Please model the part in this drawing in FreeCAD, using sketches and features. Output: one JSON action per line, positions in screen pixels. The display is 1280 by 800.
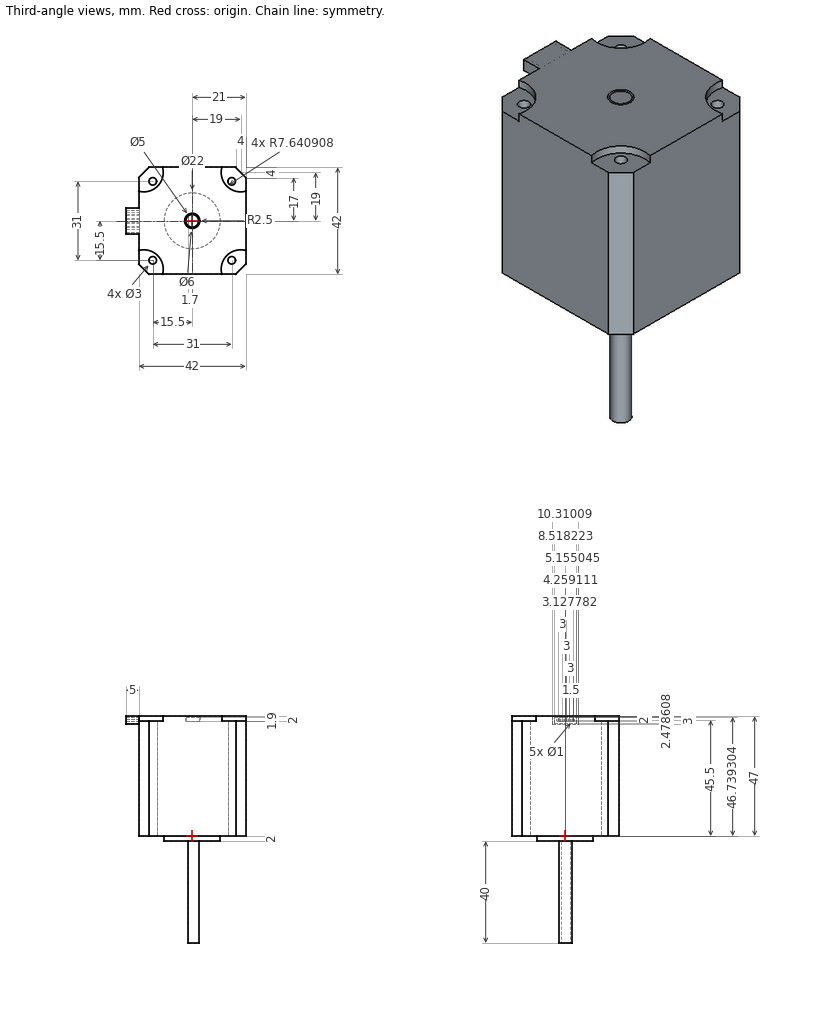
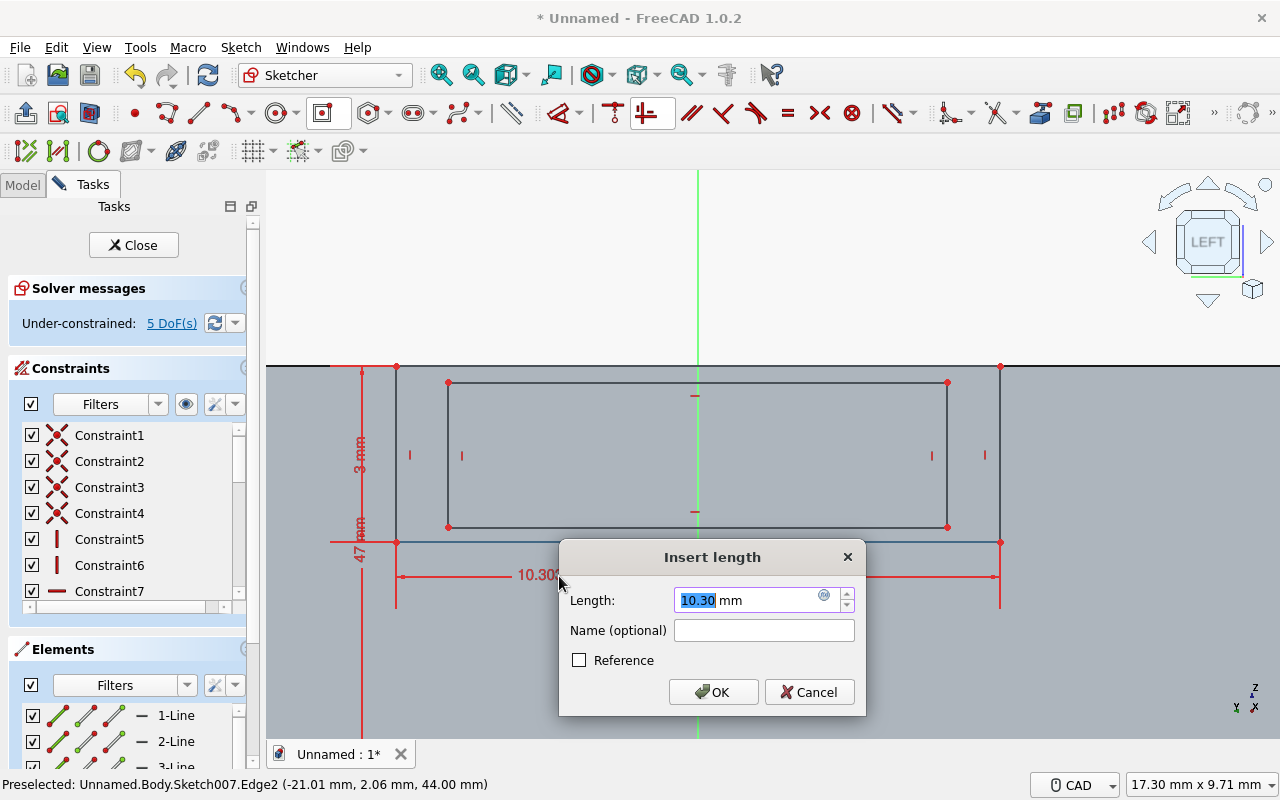
{"action": "type", "text": "10.31009"}
{"action": "key", "text": "Return"}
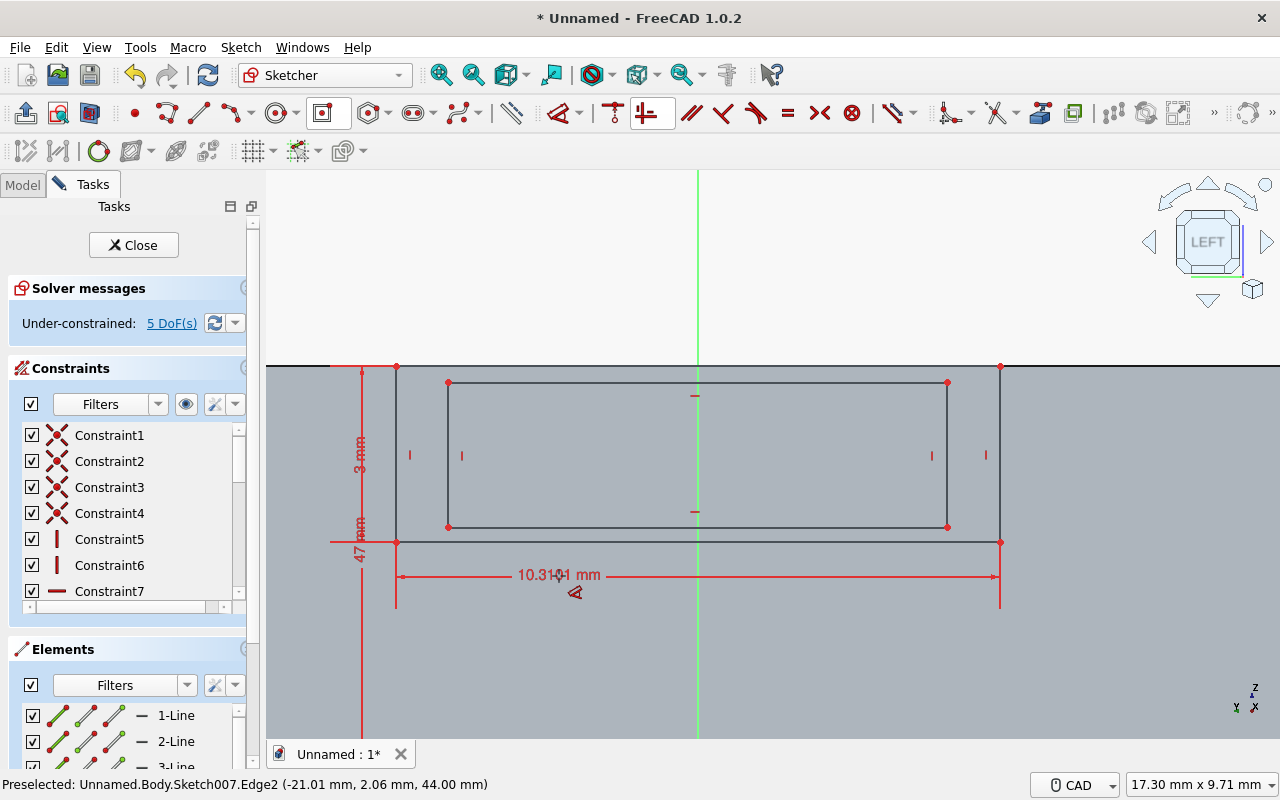
{"action": "left_click", "coordinate": [448, 427]}
{"action": "left_click", "coordinate": [414, 422]}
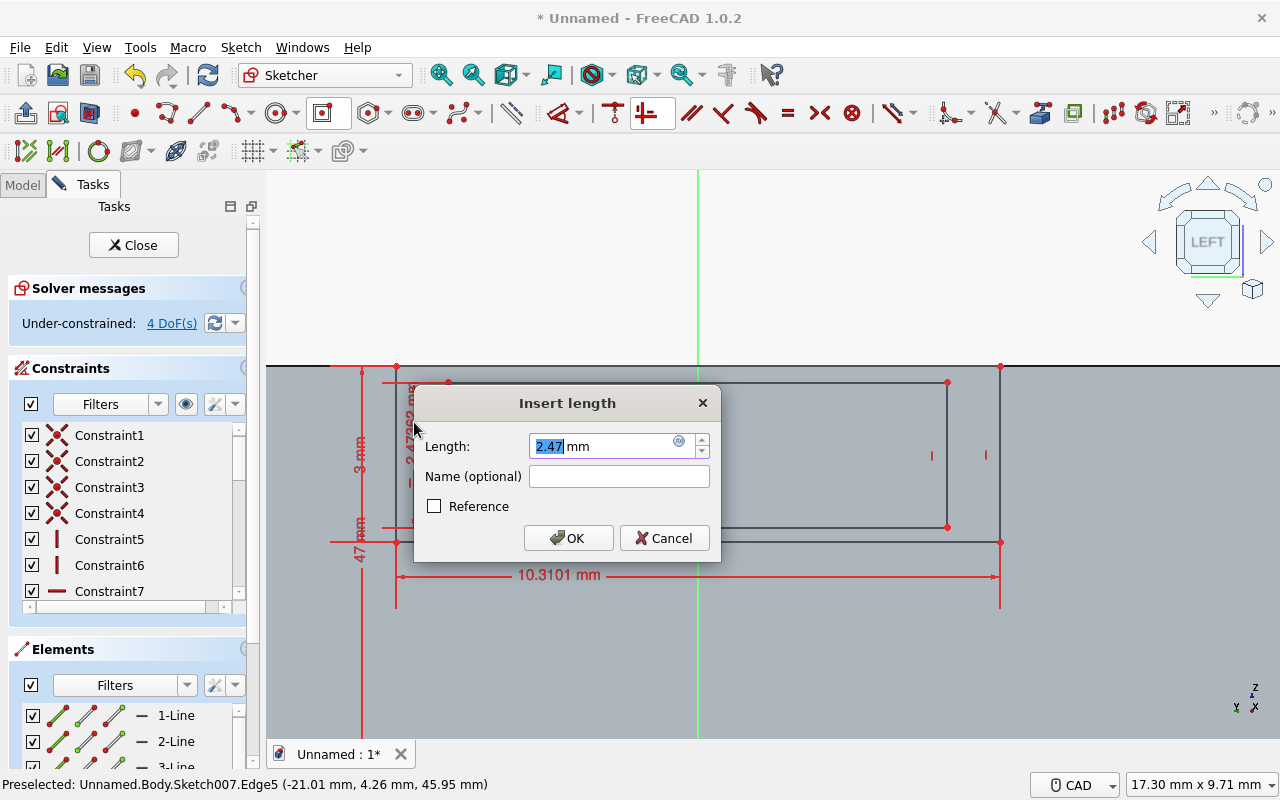
{"action": "type", "text": "2.478608"}
{"action": "key", "text": "Return"}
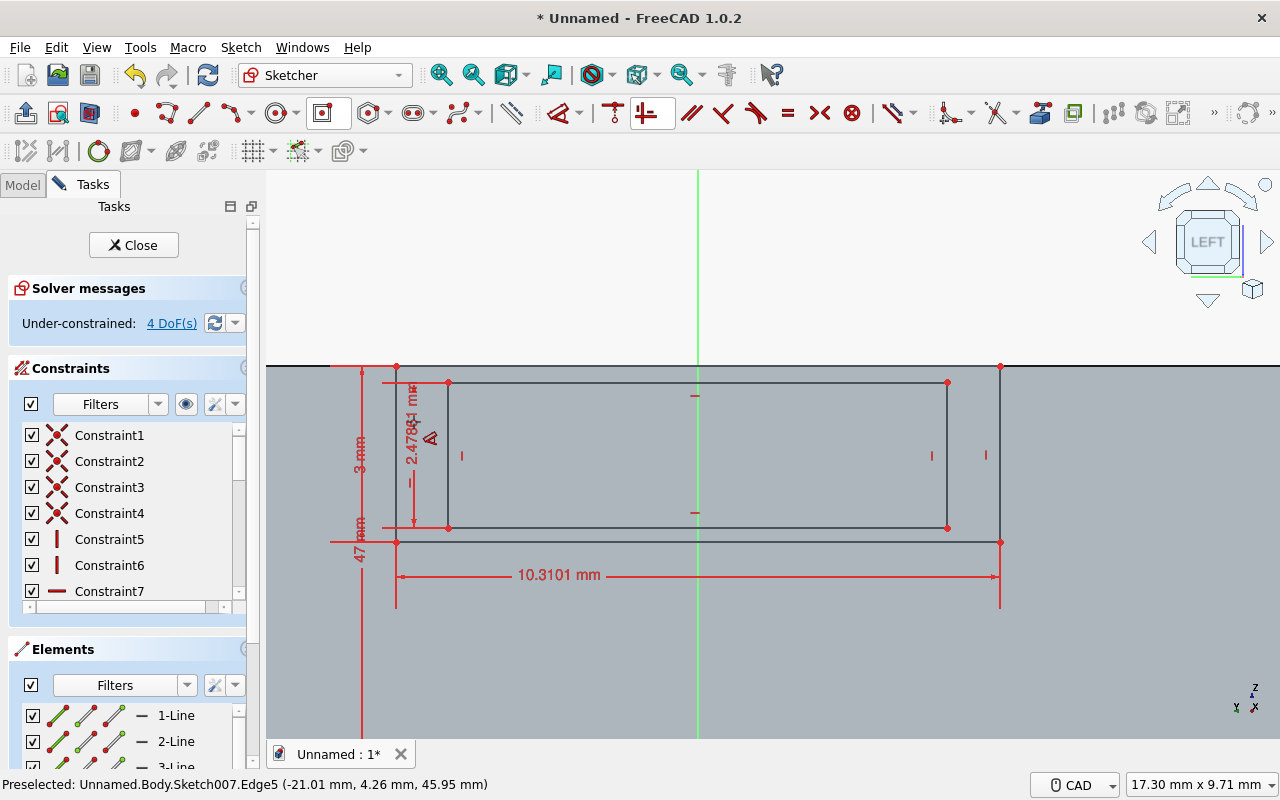
{"action": "left_click", "coordinate": [598, 528]}
{"action": "left_click", "coordinate": [812, 562]}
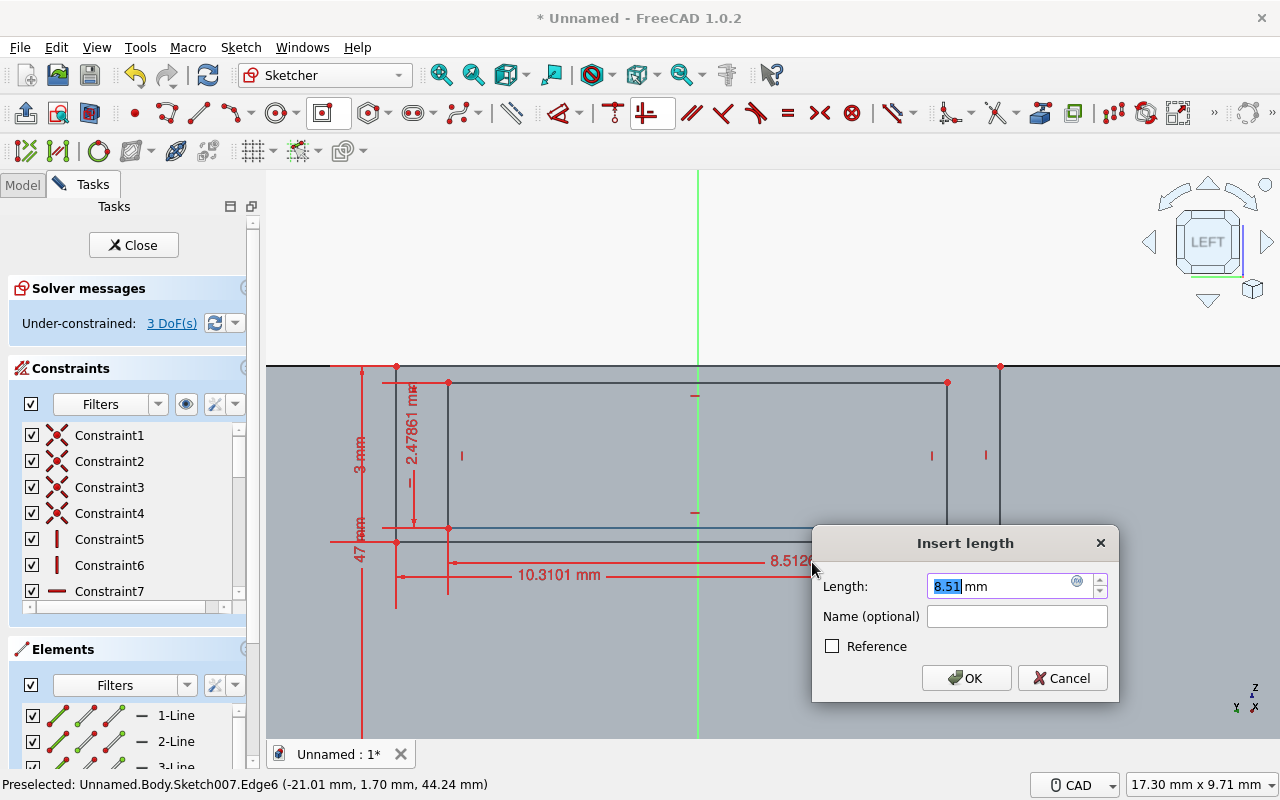
{"action": "type", "text": "8.518223"}
{"action": "key", "text": "Return"}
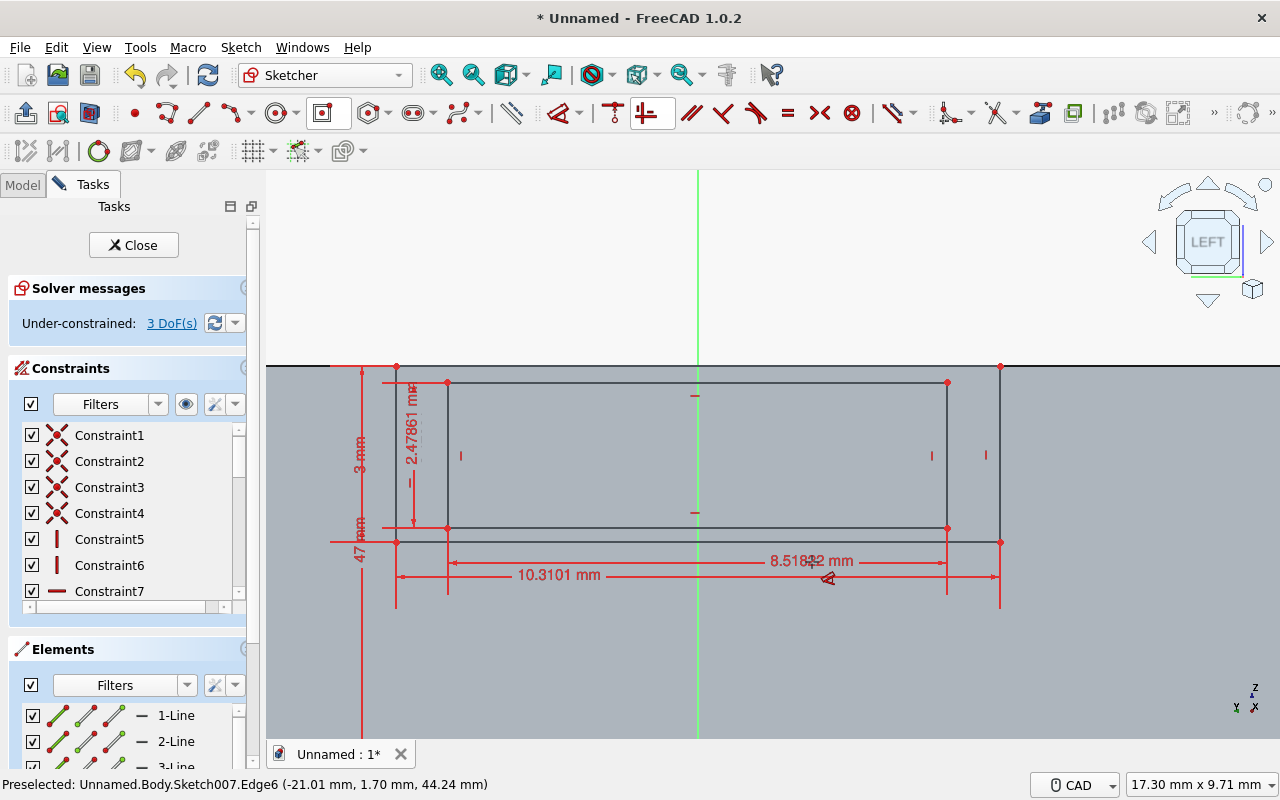
{"action": "left_click", "coordinate": [396, 366]}
{"action": "left_click", "coordinate": [547, 332]}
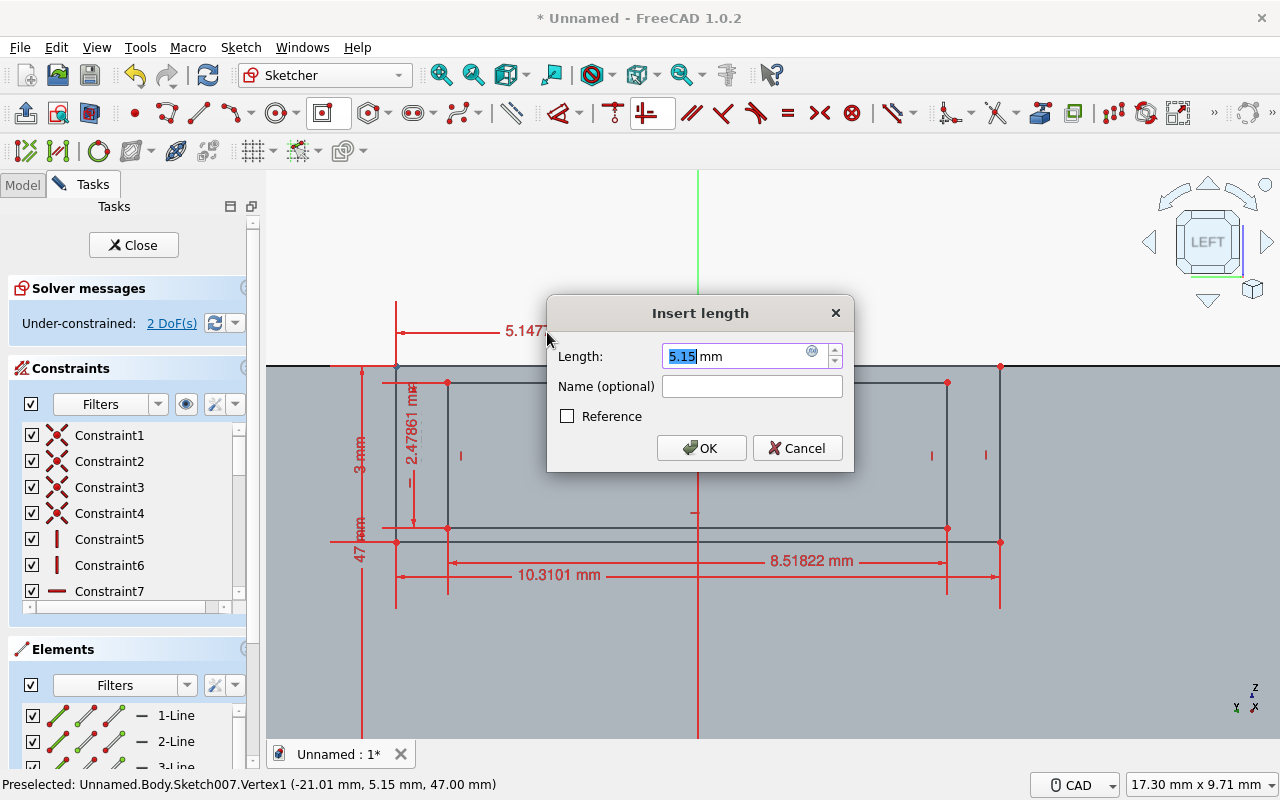
{"action": "type", "text": "5.155045"}
{"action": "key", "text": "Return"}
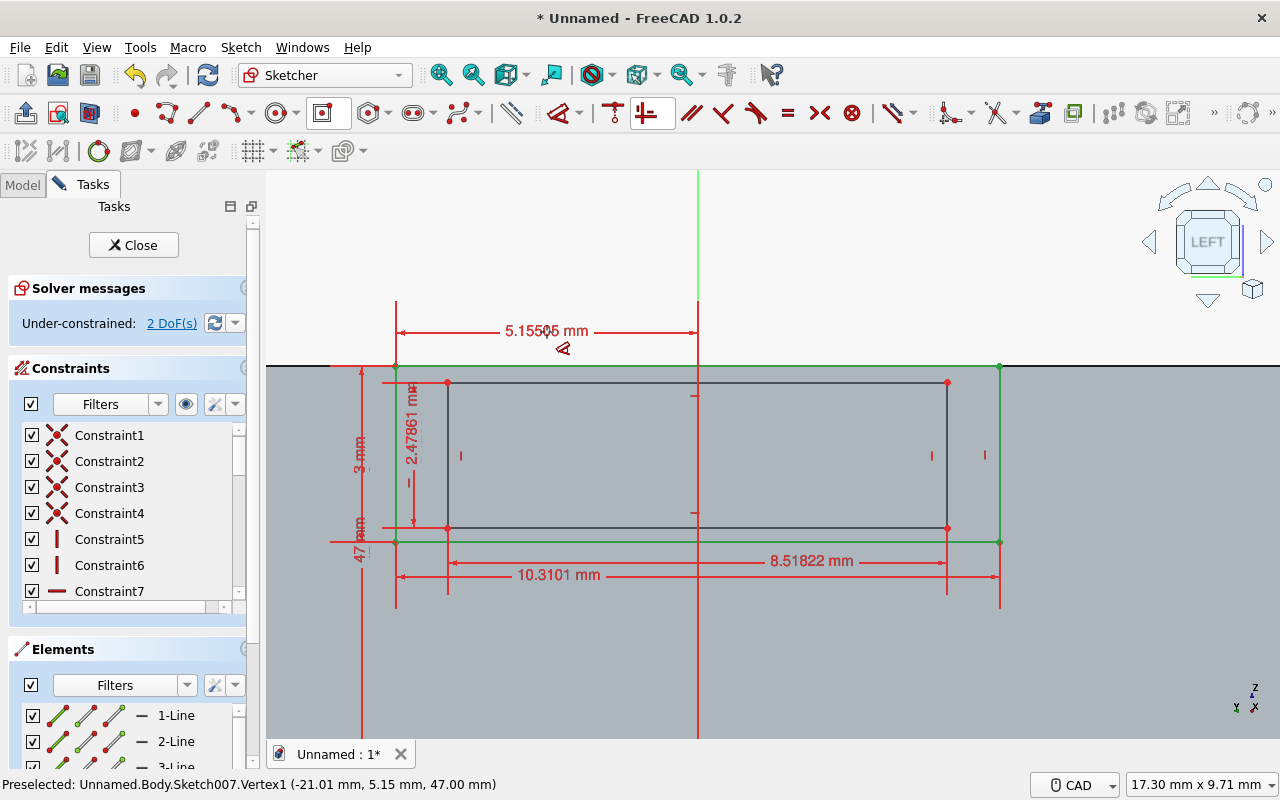
{"action": "left_click", "coordinate": [448, 383]}
{"action": "left_click", "coordinate": [630, 349]}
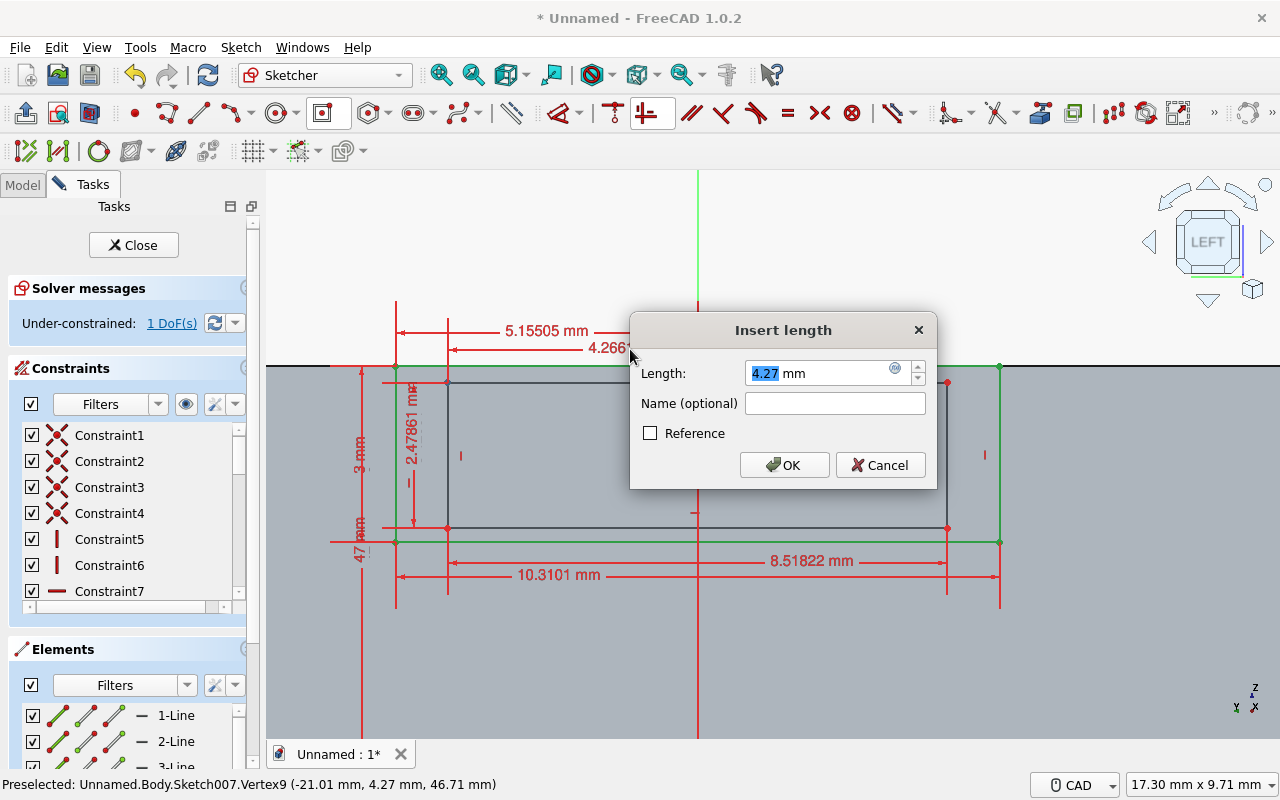
{"action": "type", "text": "4.259111"}
{"action": "key", "text": "Return"}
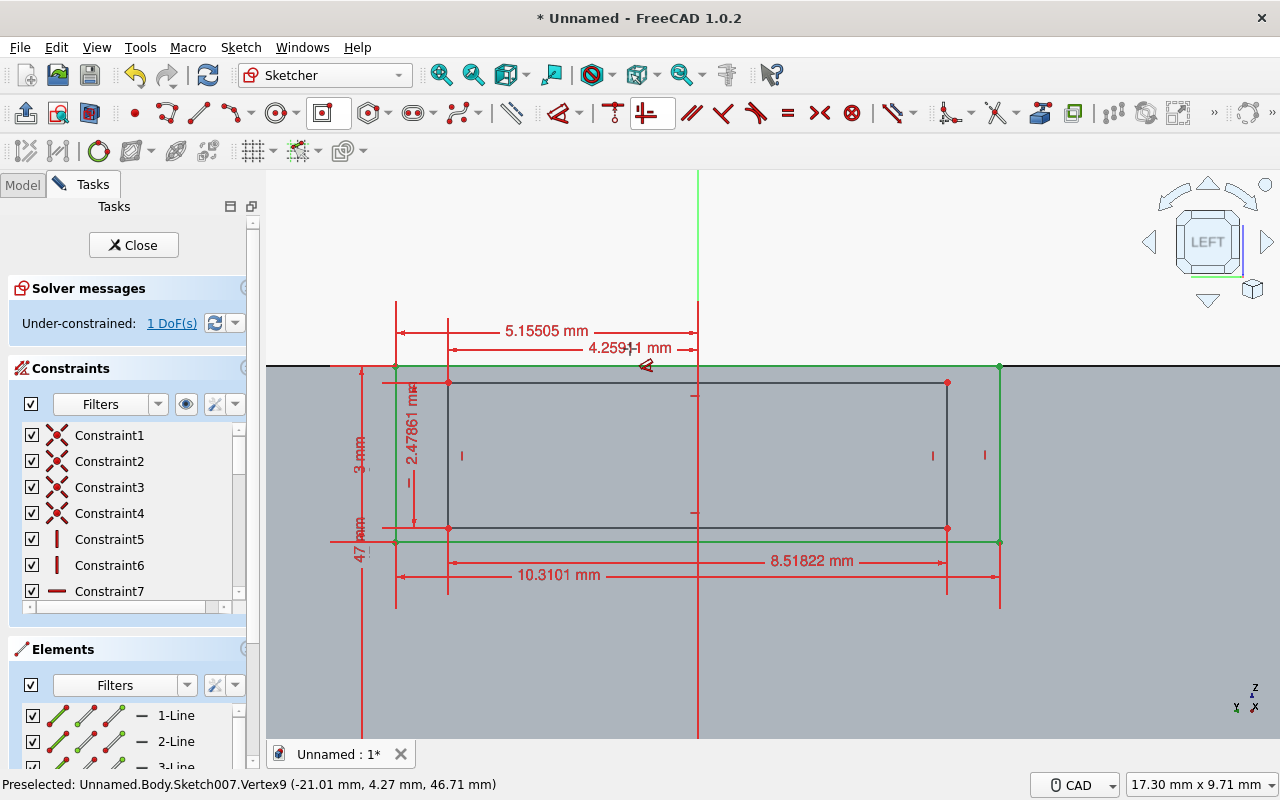
{"action": "left_click", "coordinate": [448, 383]}
{"action": "left_click", "coordinate": [414, 622]}